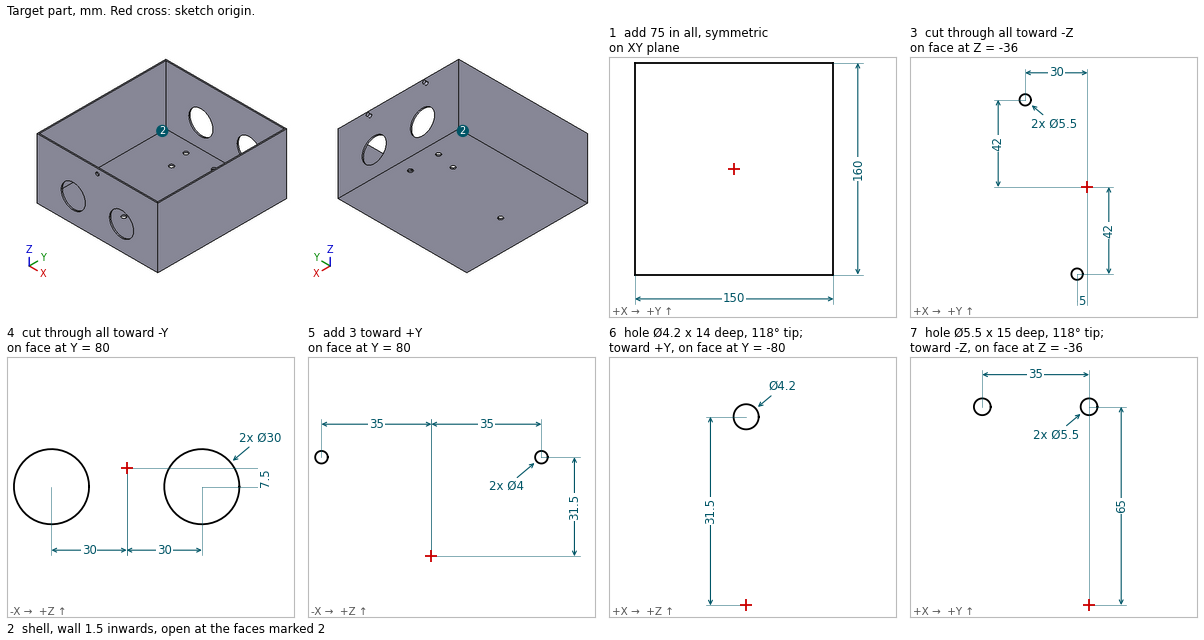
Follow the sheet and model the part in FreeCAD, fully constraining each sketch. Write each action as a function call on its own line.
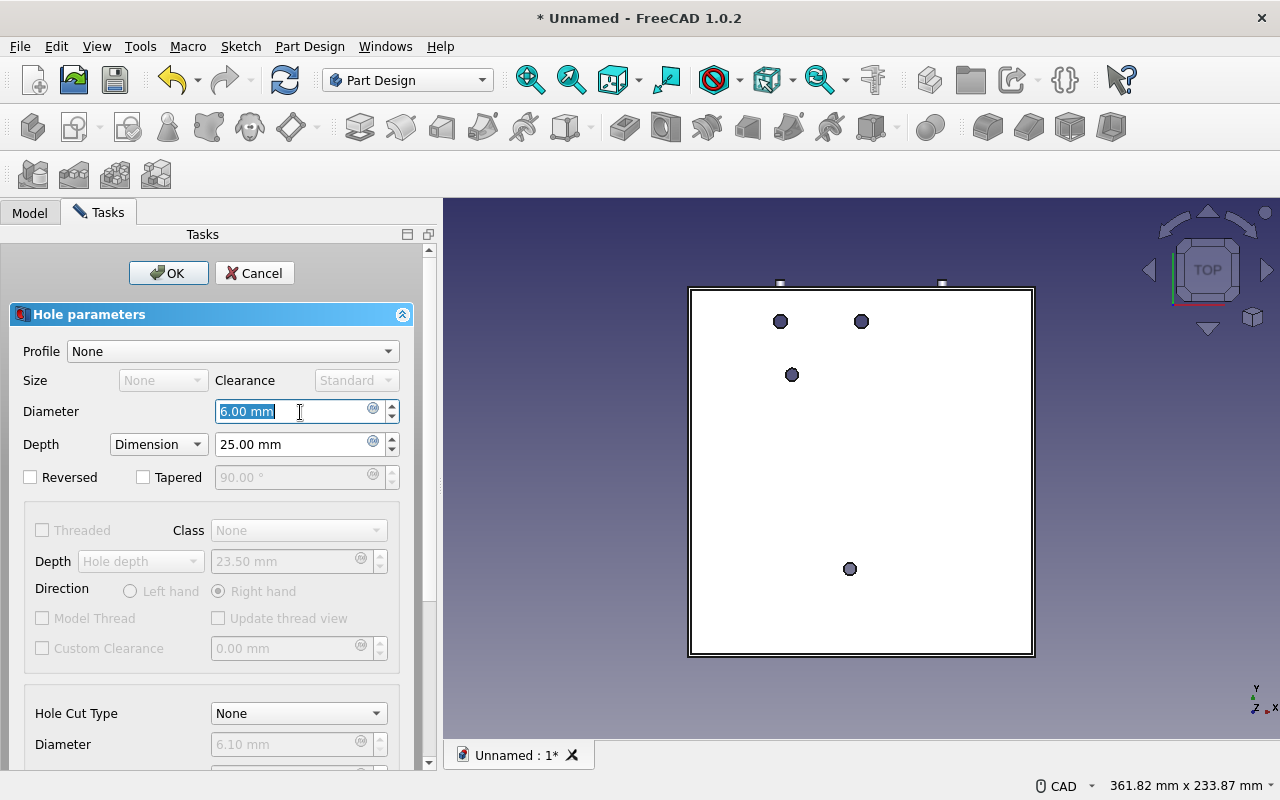
text(5.5)
key(Tab)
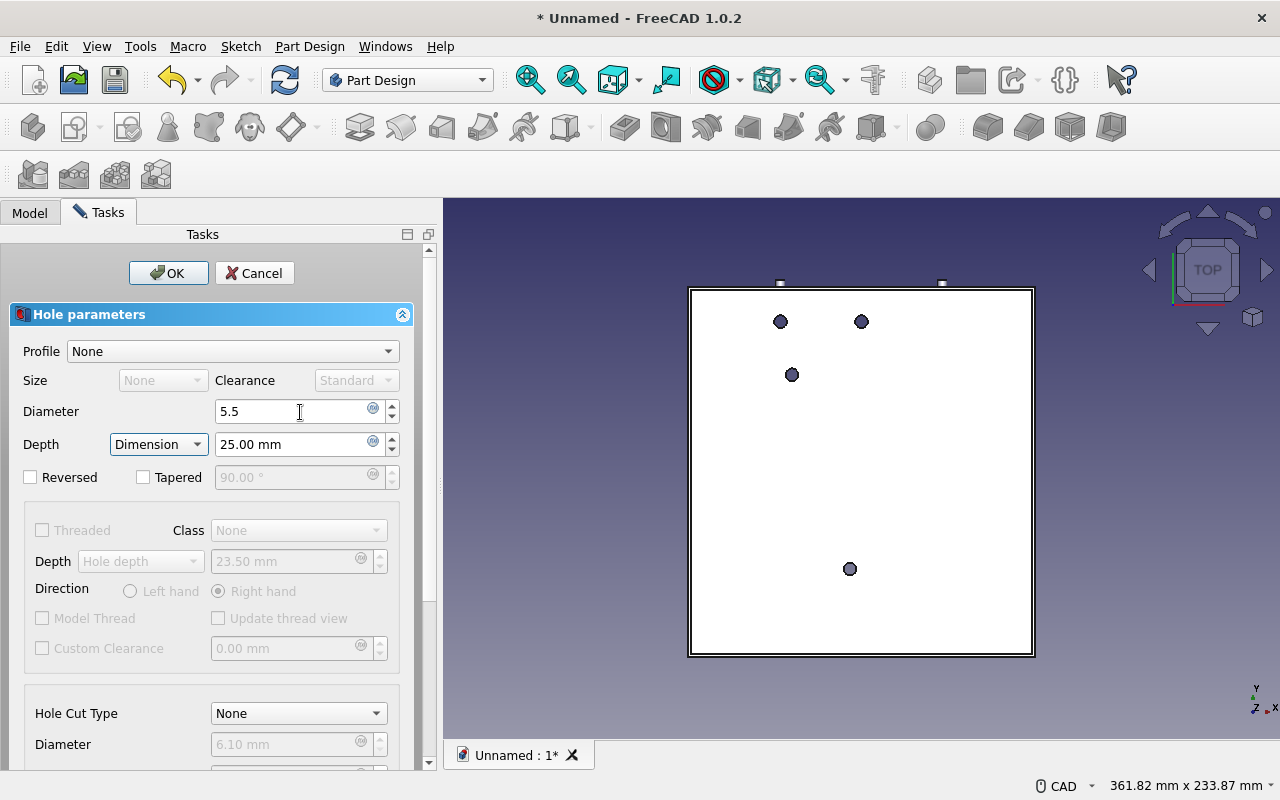
triple_click(300, 444)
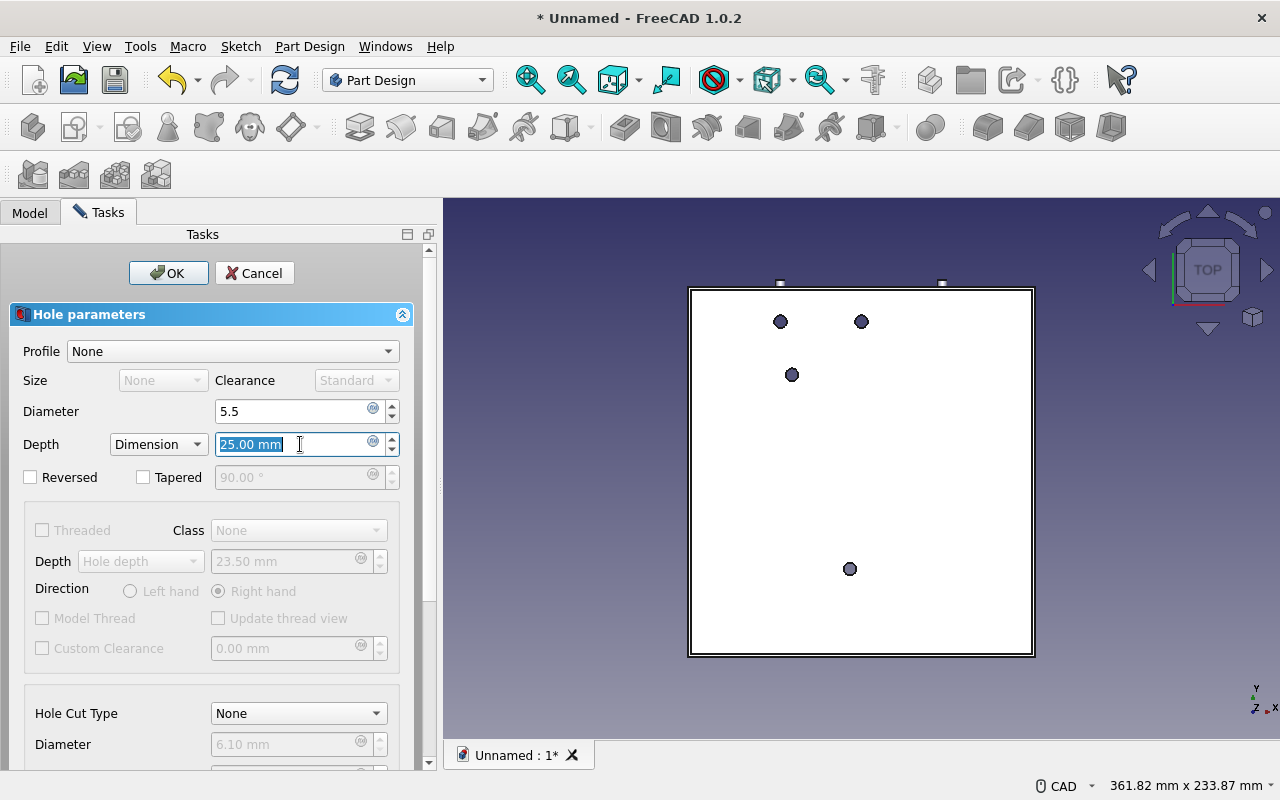
text(15)
key(Tab)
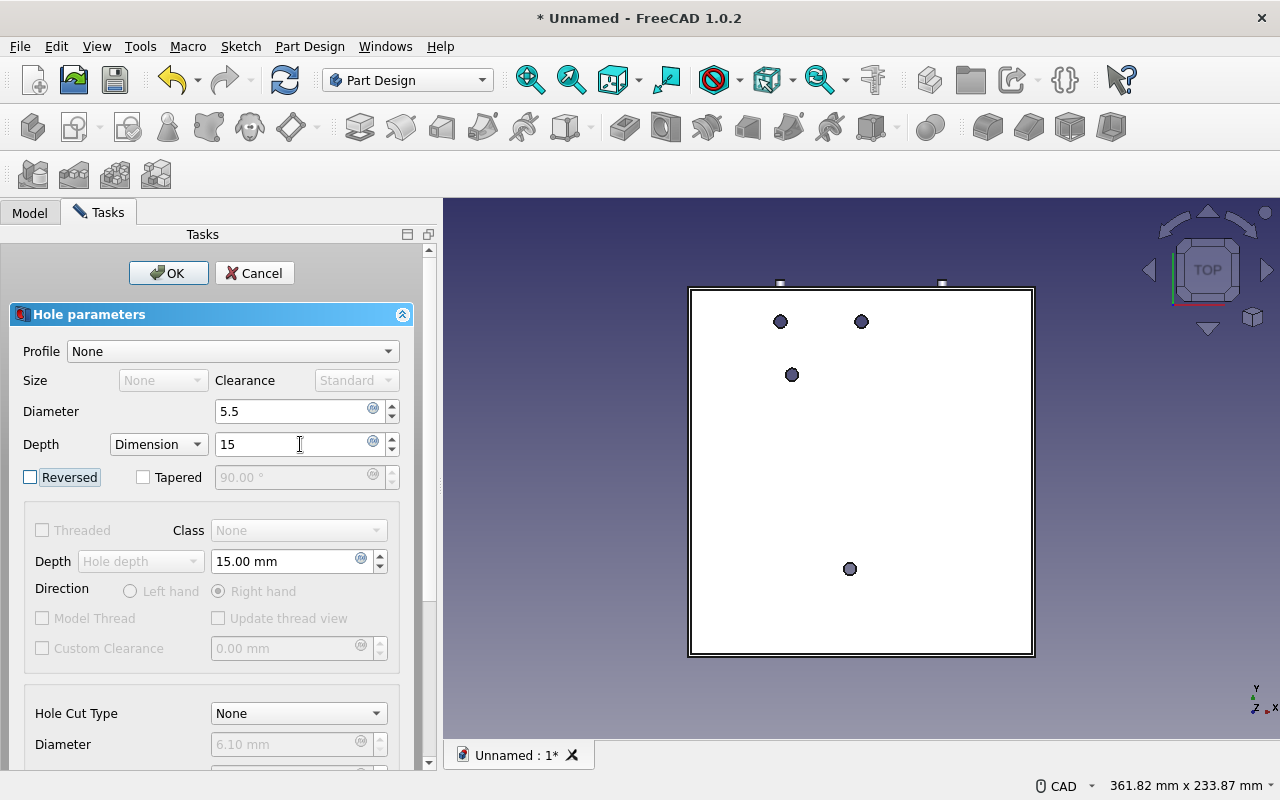
click(169, 273)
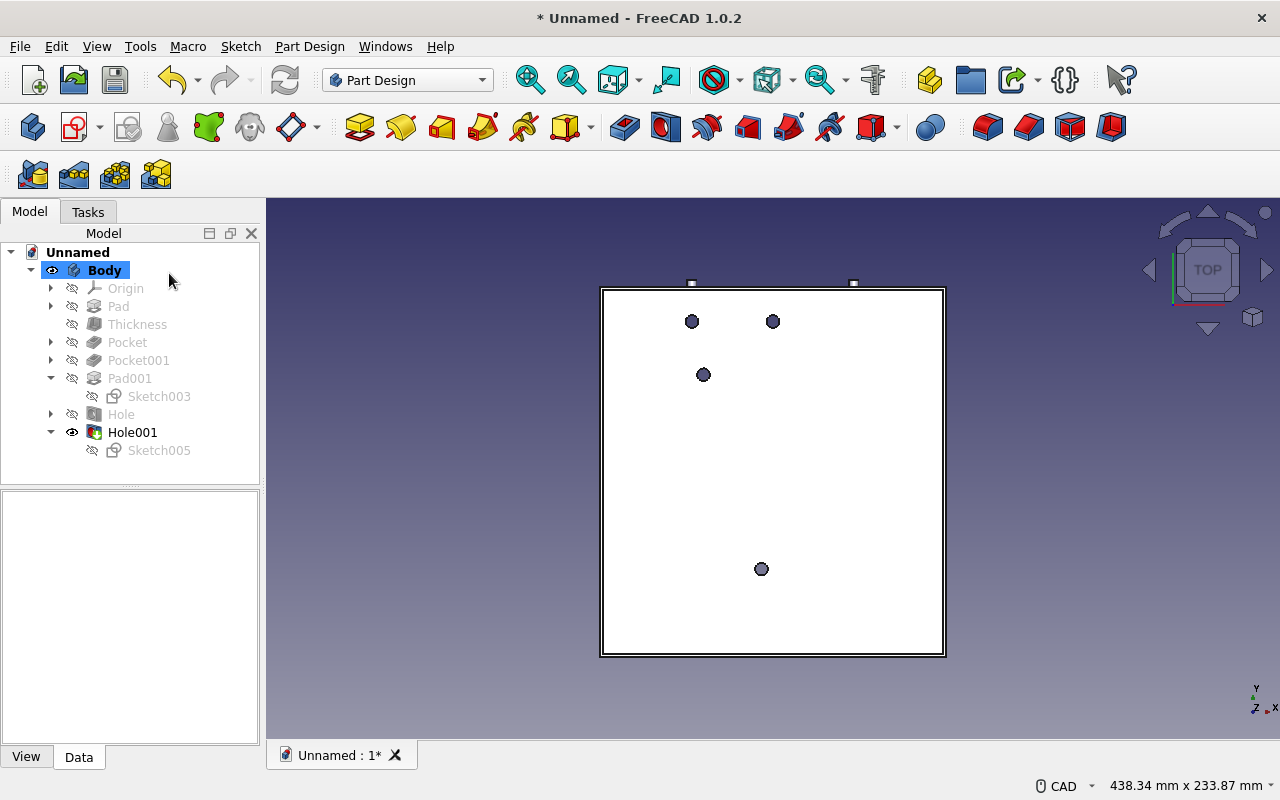
key(0)